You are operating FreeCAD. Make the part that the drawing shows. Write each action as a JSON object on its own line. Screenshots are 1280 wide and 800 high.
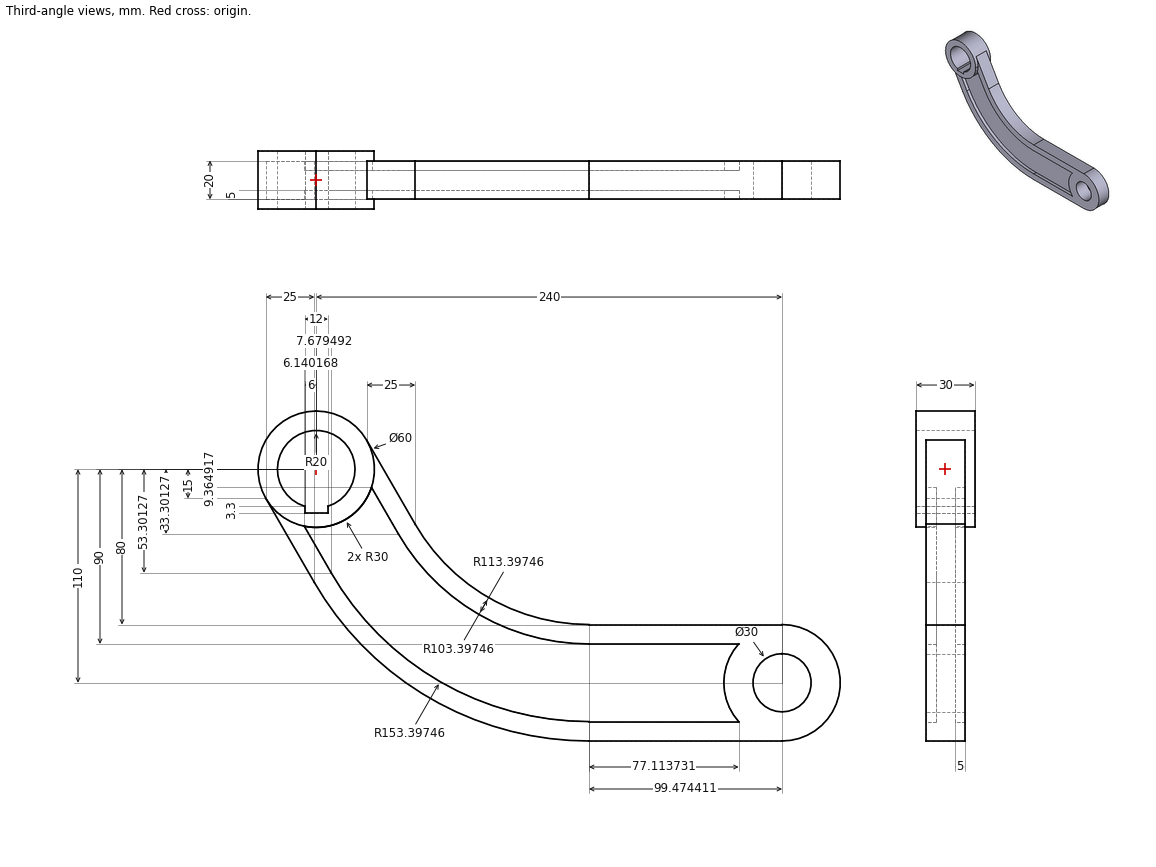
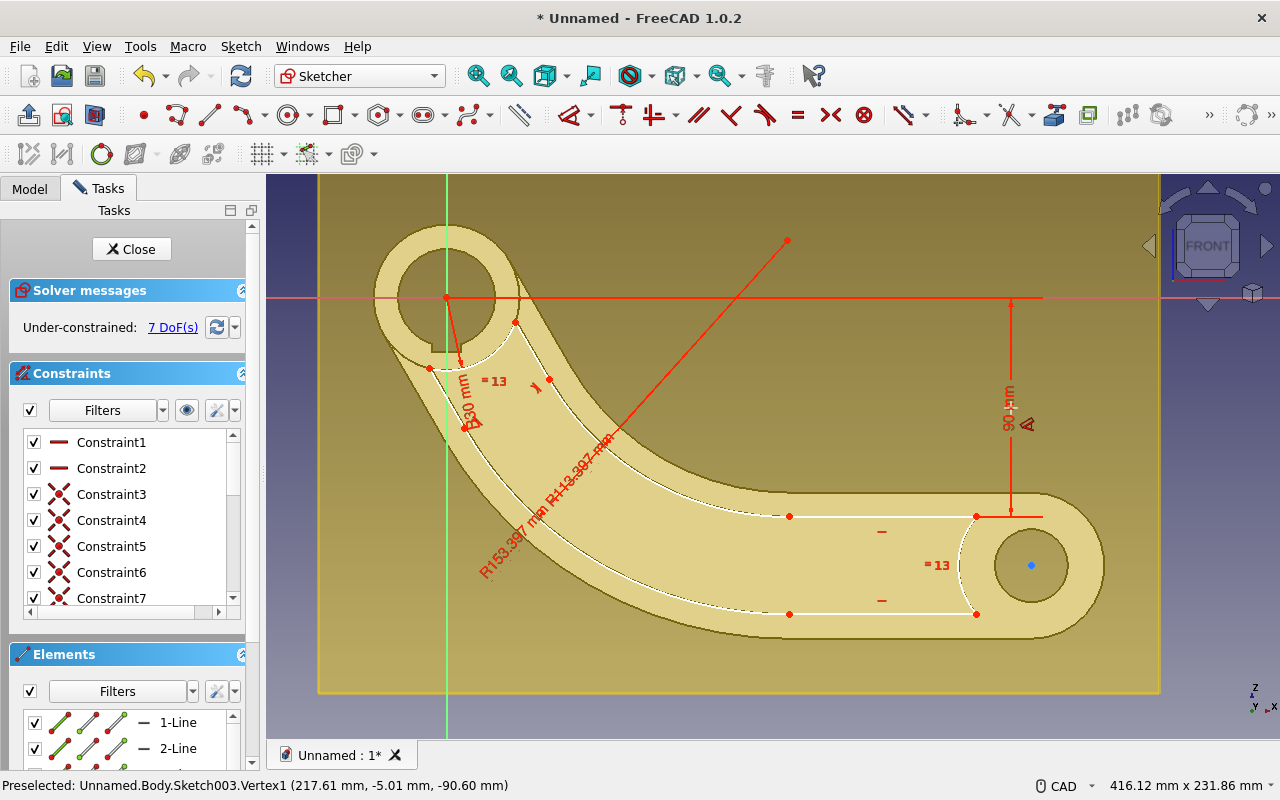
{"action": "left_click", "coordinate": [1031, 566]}
{"action": "left_click", "coordinate": [739, 264]}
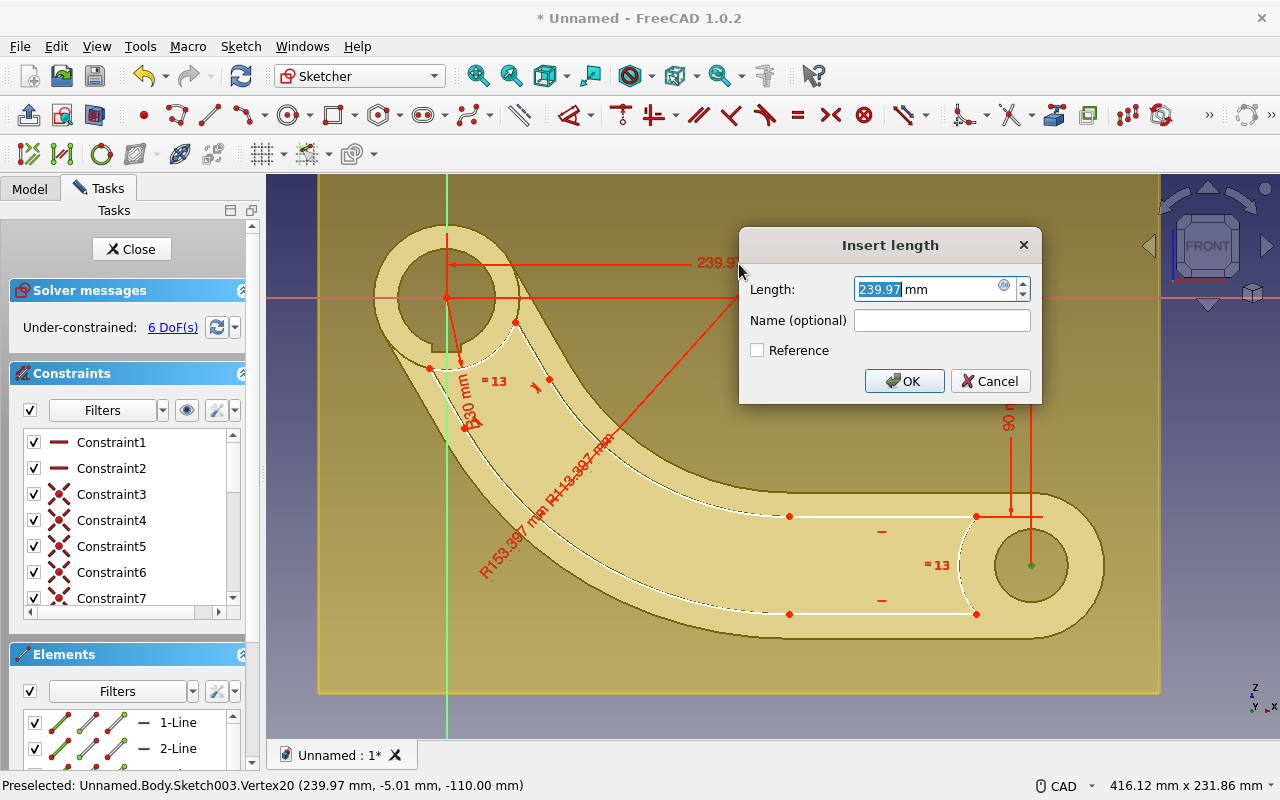
{"action": "type", "text": "240"}
{"action": "key", "text": "Return"}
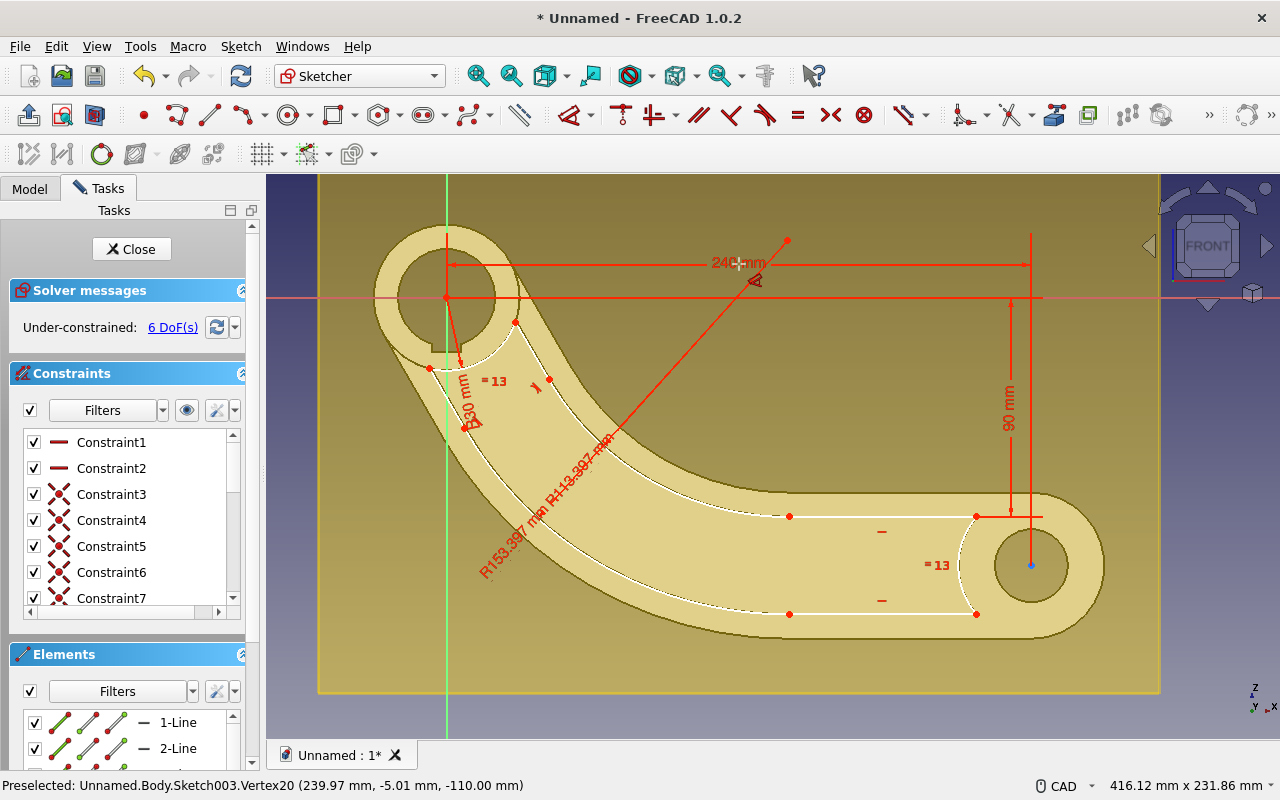
{"action": "left_click", "coordinate": [1031, 566]}
{"action": "left_click", "coordinate": [1065, 432]}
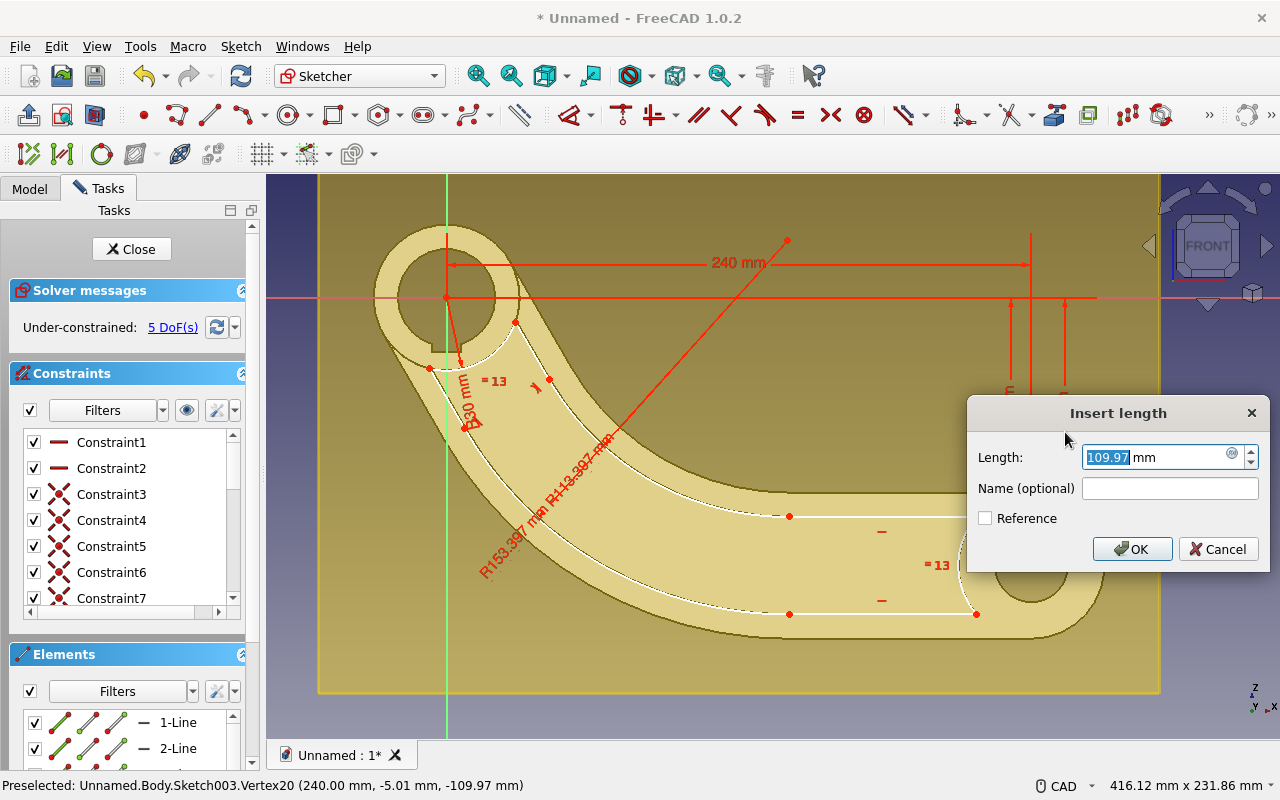
{"action": "type", "text": "110"}
{"action": "key", "text": "Return"}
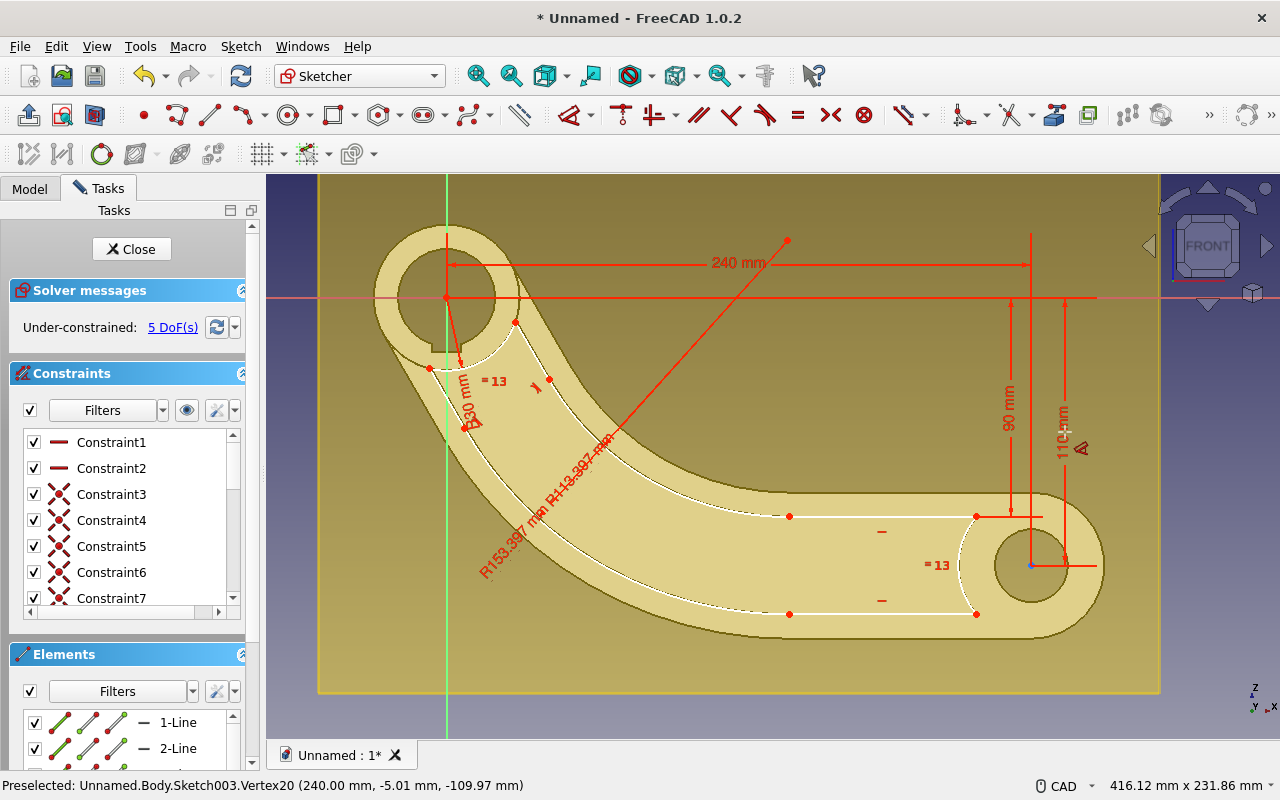
{"action": "left_click", "coordinate": [921, 517]}
{"action": "left_click", "coordinate": [883, 551]}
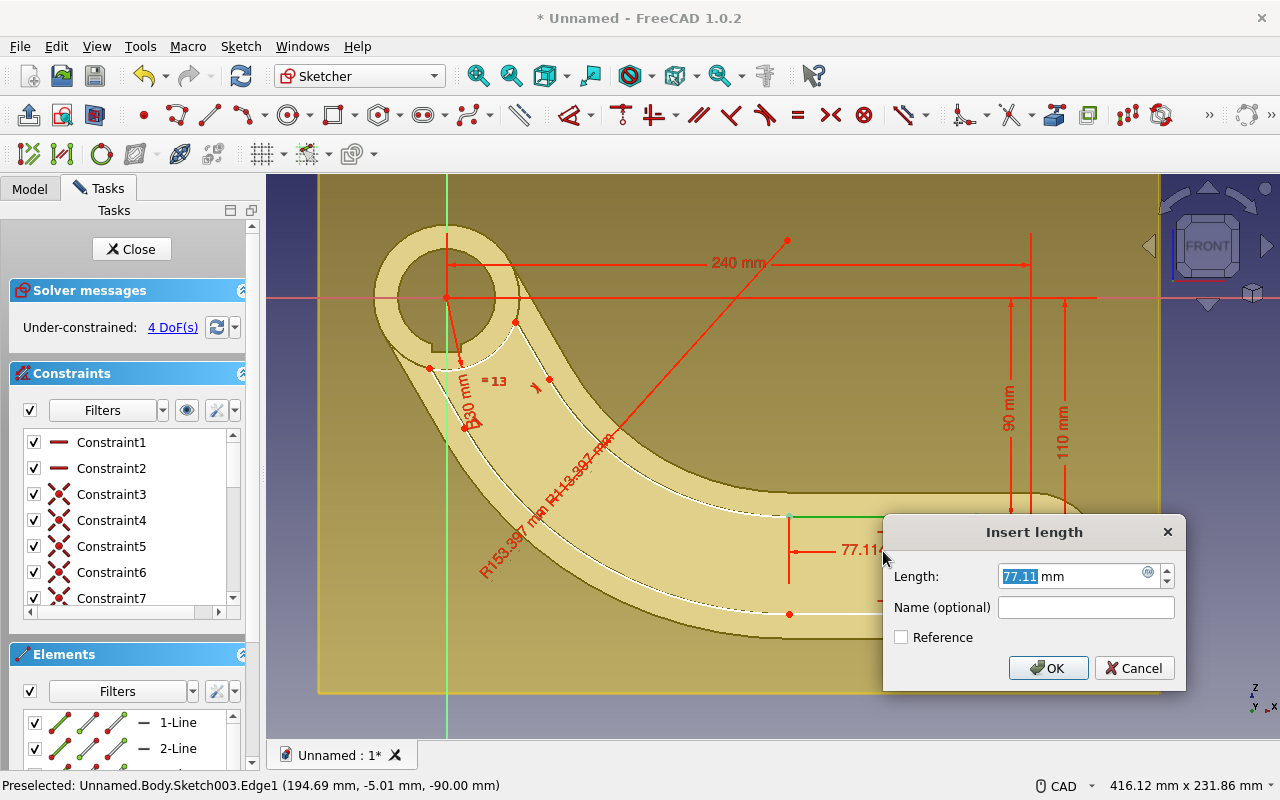
{"action": "type", "text": "77.113731"}
{"action": "key", "text": "Return"}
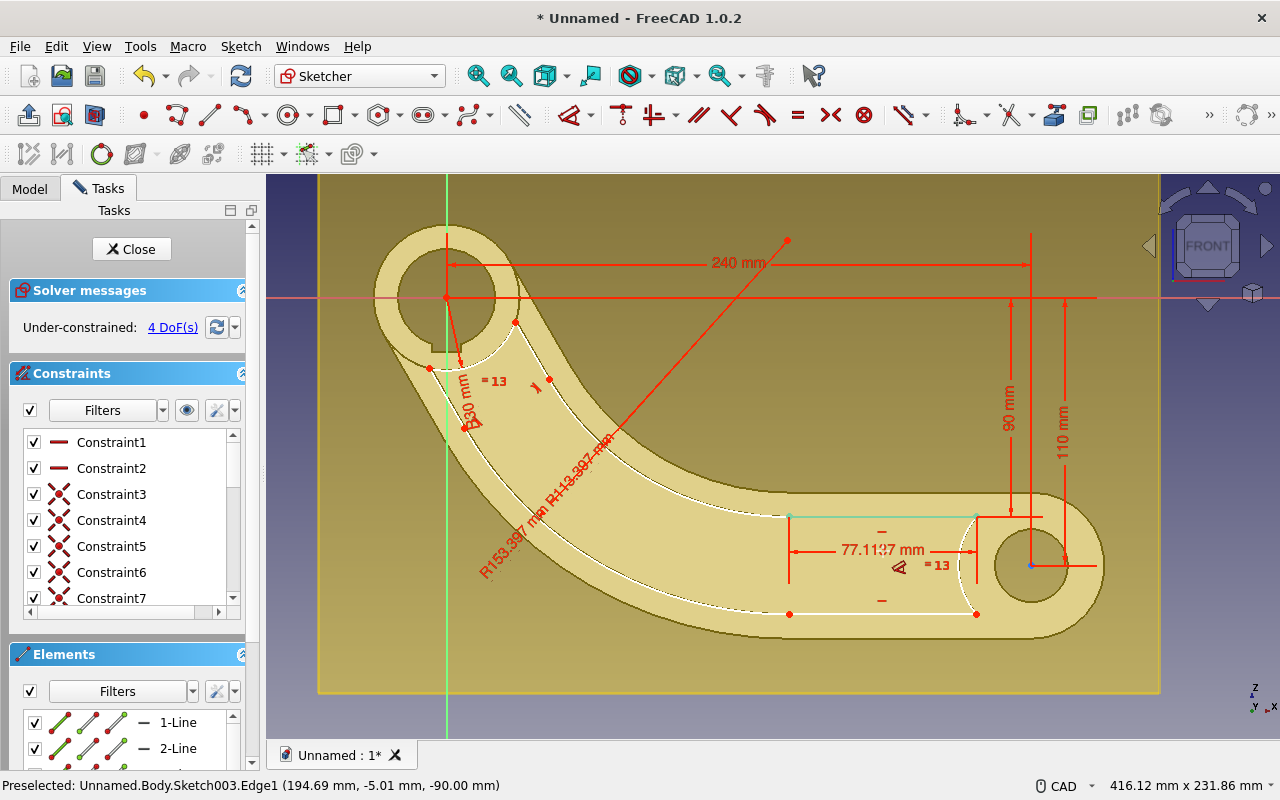
{"action": "left_click", "coordinate": [845, 614]}
{"action": "left_click", "coordinate": [883, 648]}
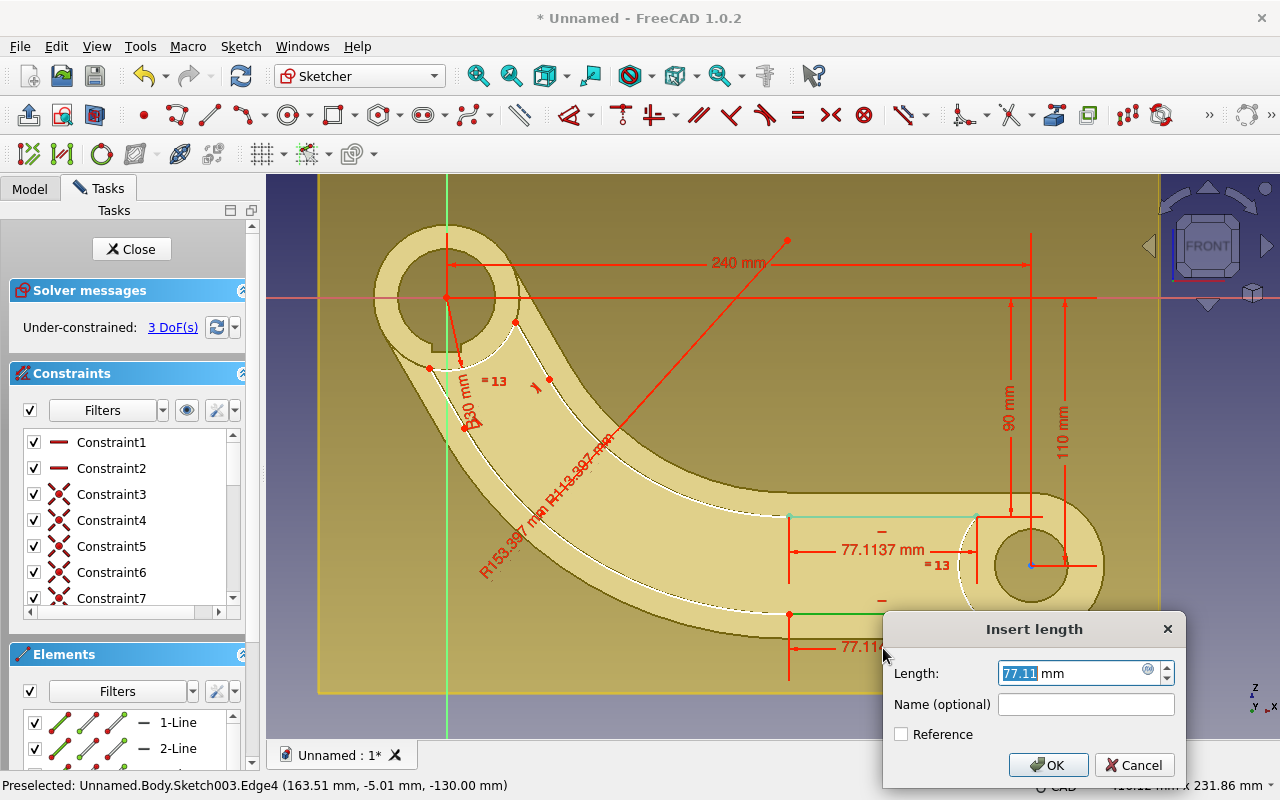
{"action": "type", "text": "77.113731"}
{"action": "key", "text": "Return"}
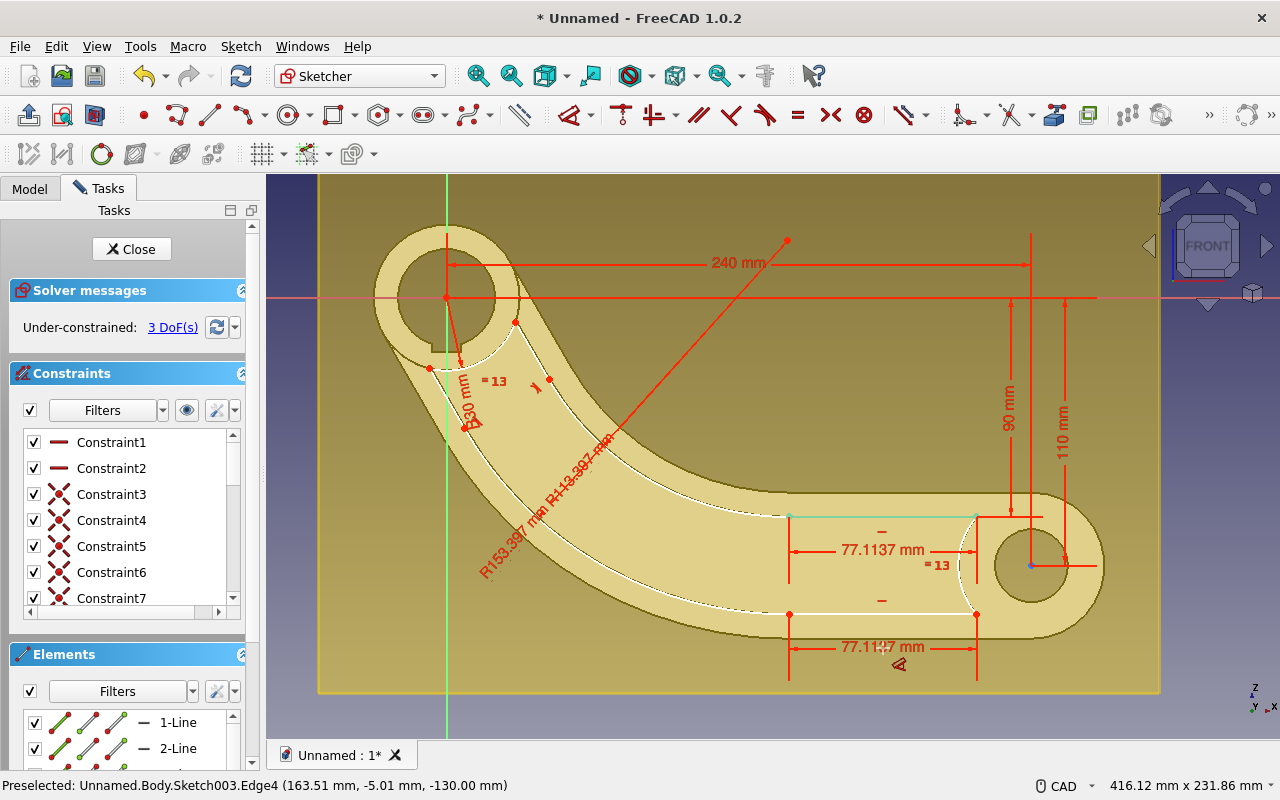
{"action": "left_click", "coordinate": [549, 380]}
{"action": "left_click", "coordinate": [413, 339]}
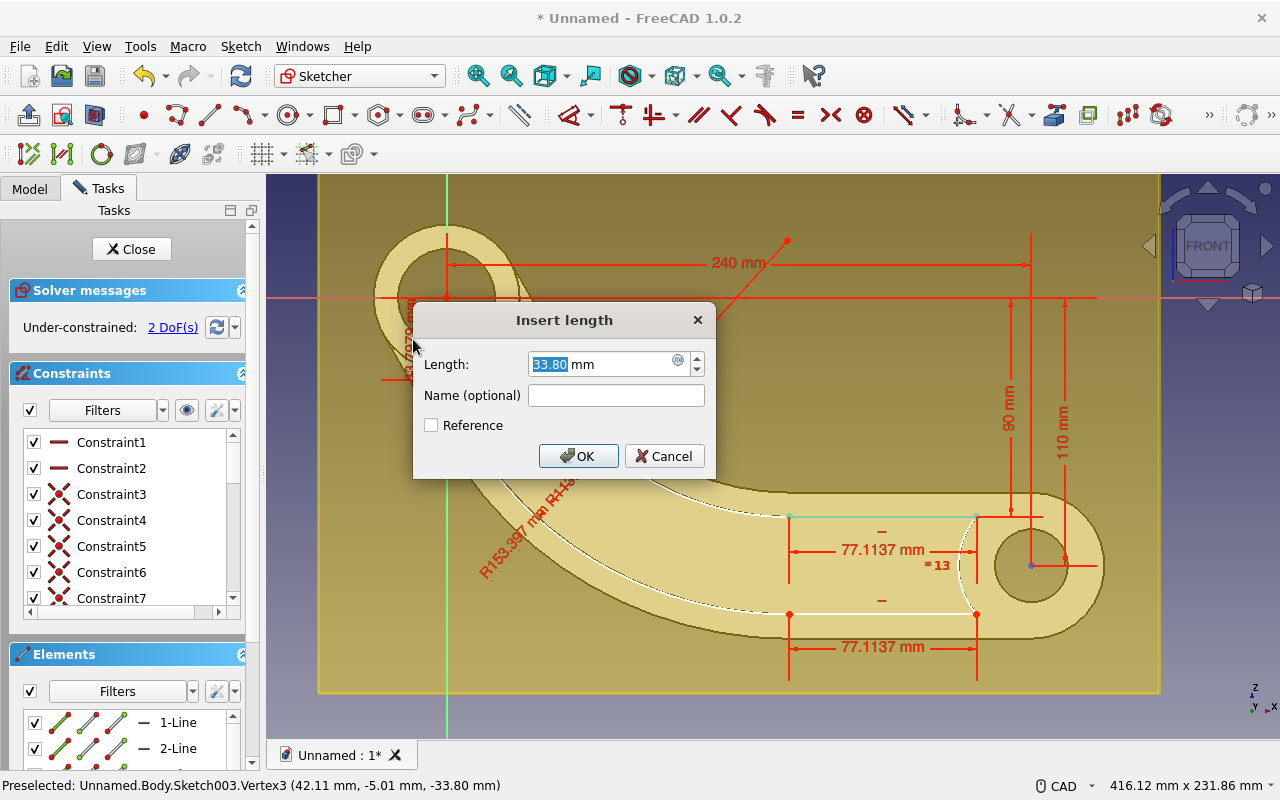
{"action": "type", "text": "33.30127"}
{"action": "key", "text": "Return"}